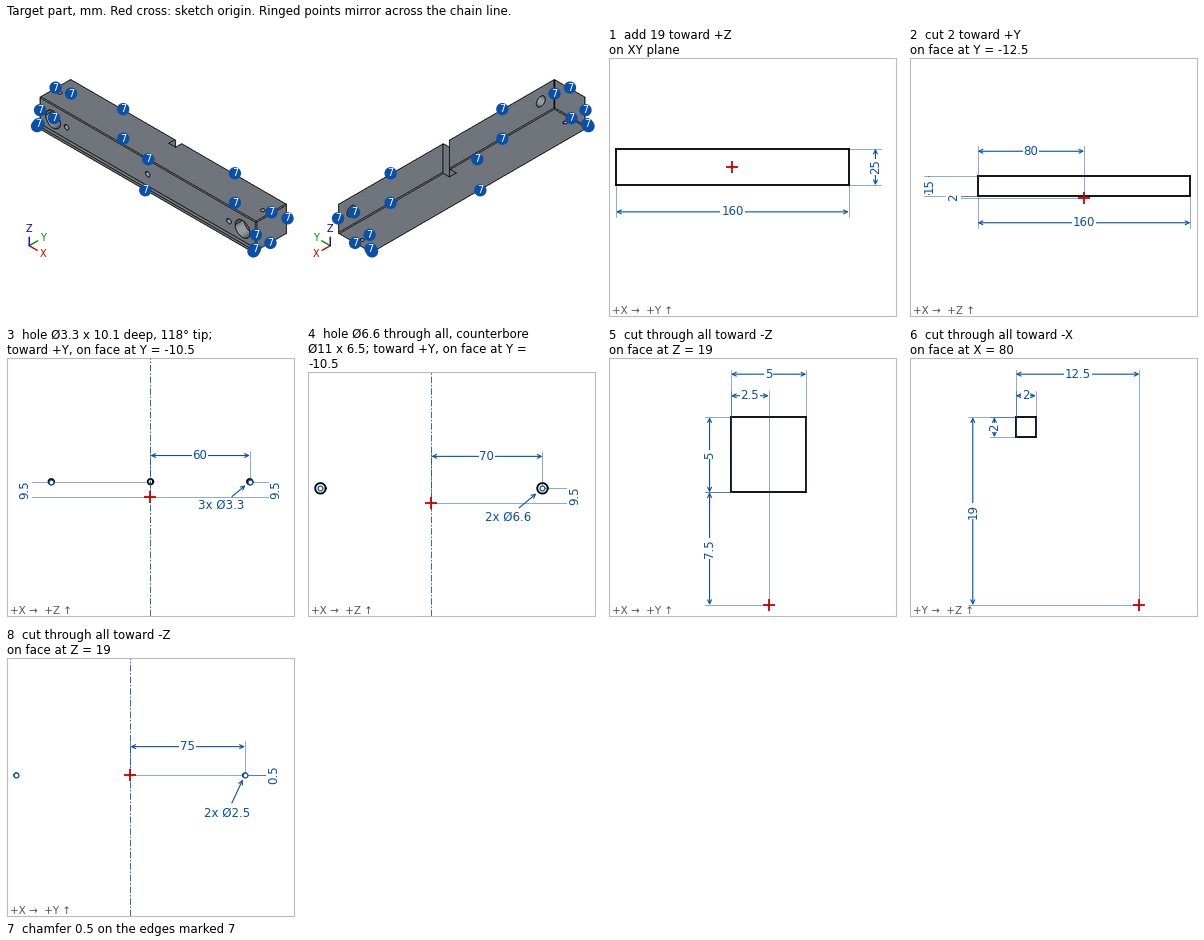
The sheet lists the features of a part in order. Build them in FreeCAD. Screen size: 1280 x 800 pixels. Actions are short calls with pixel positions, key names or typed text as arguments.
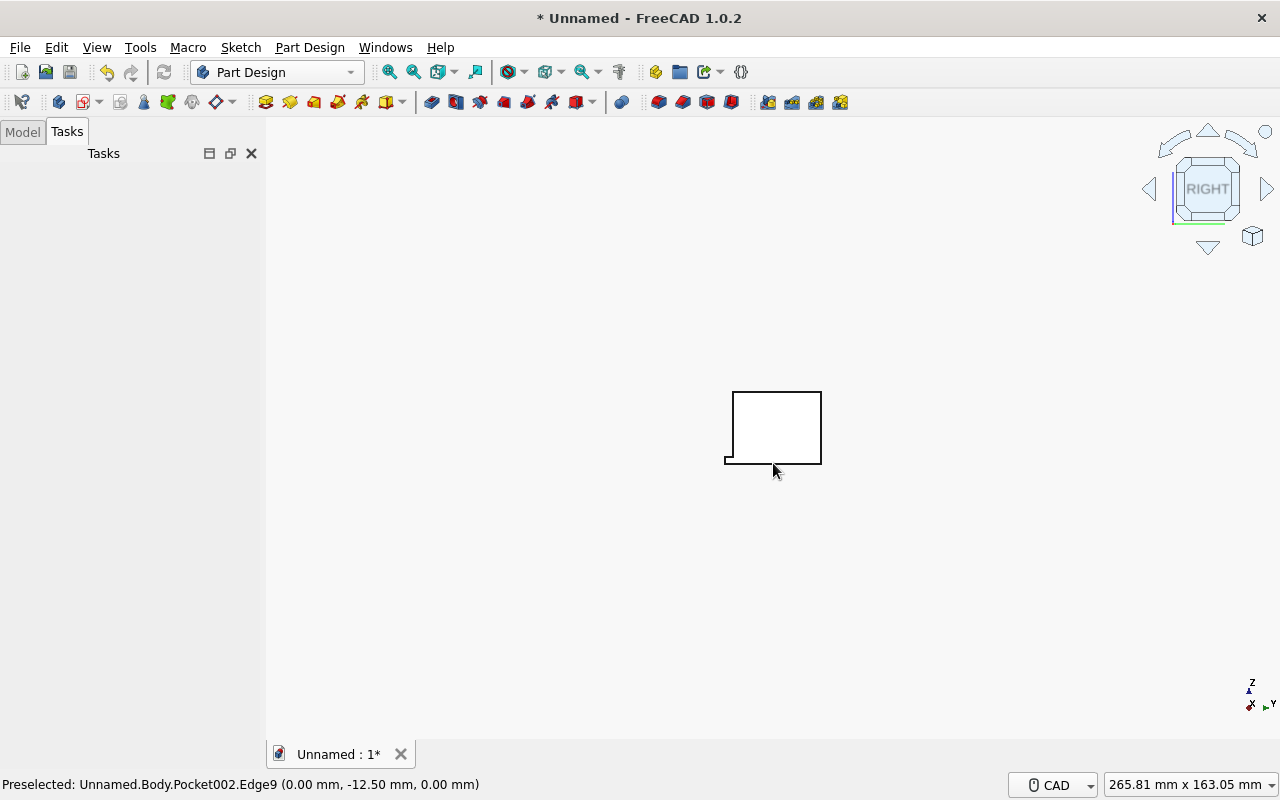
click(390, 72)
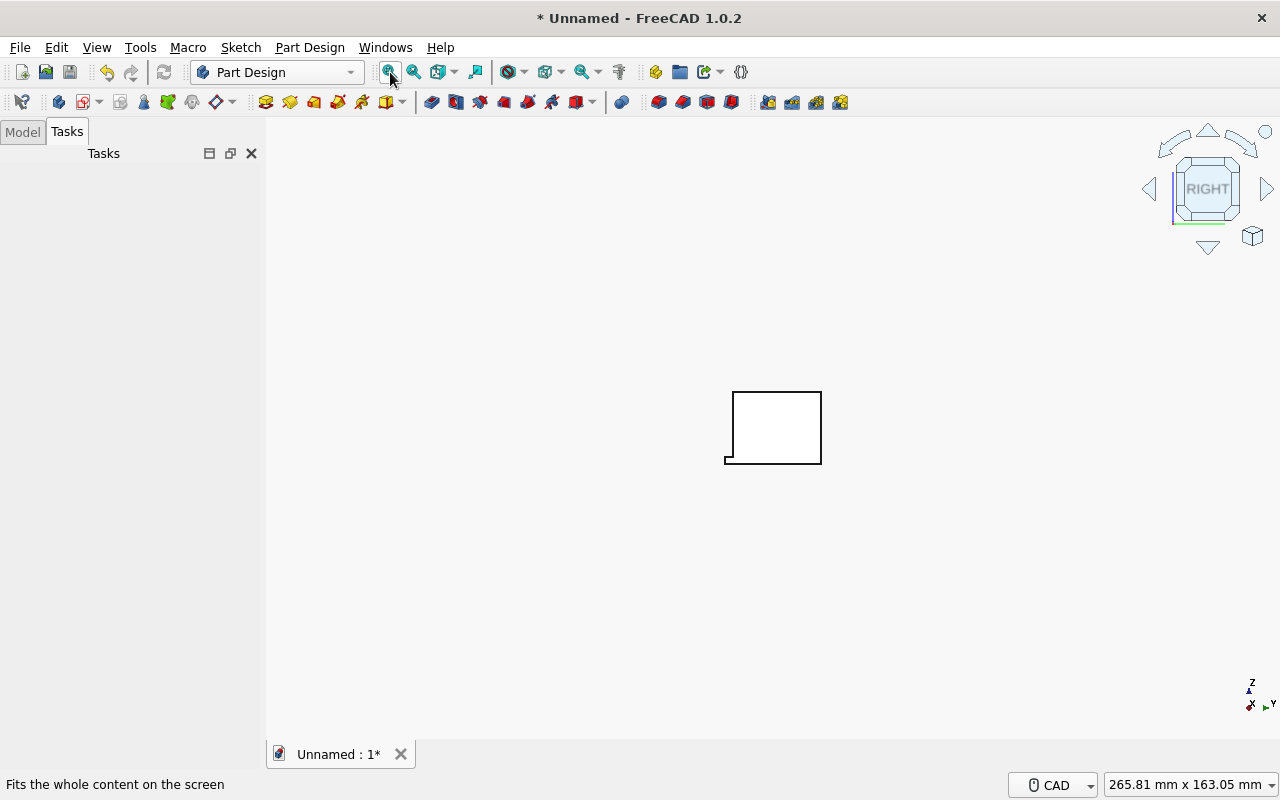
key(5)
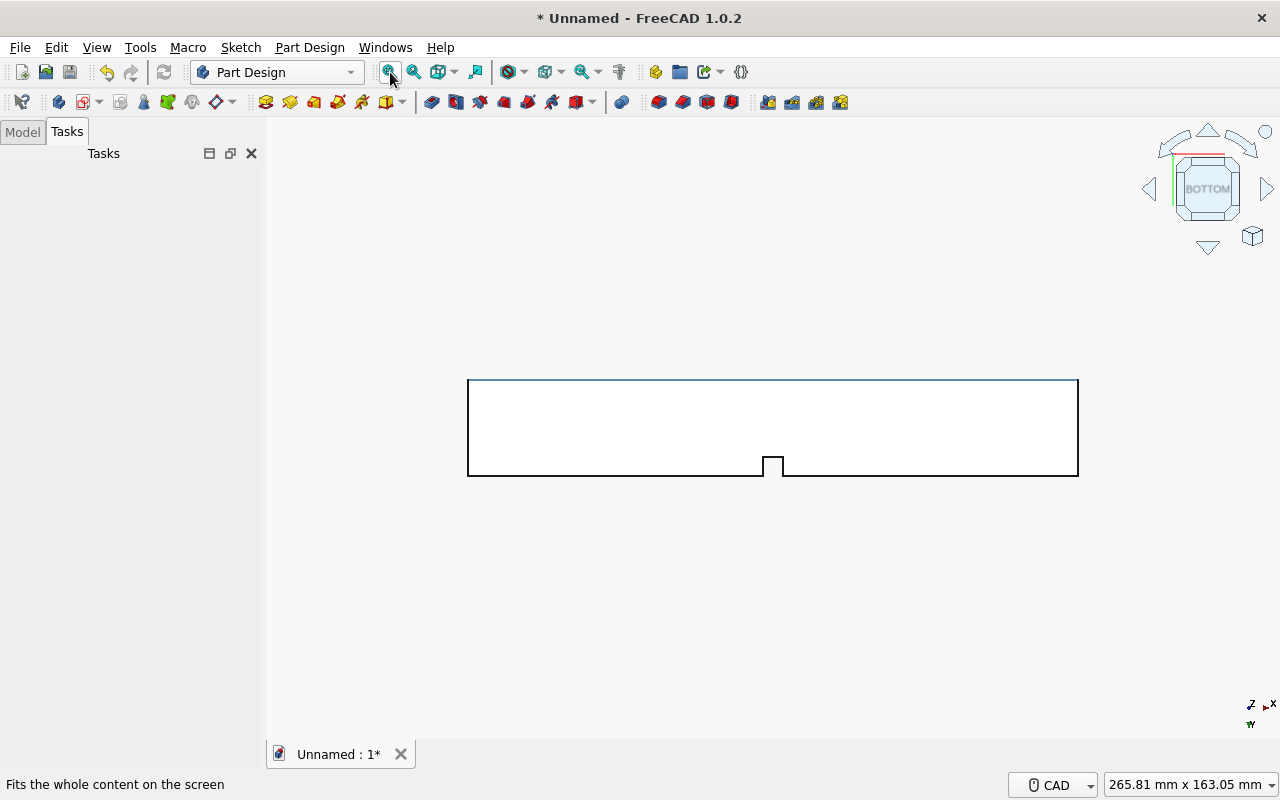
click(930, 475, ctrl)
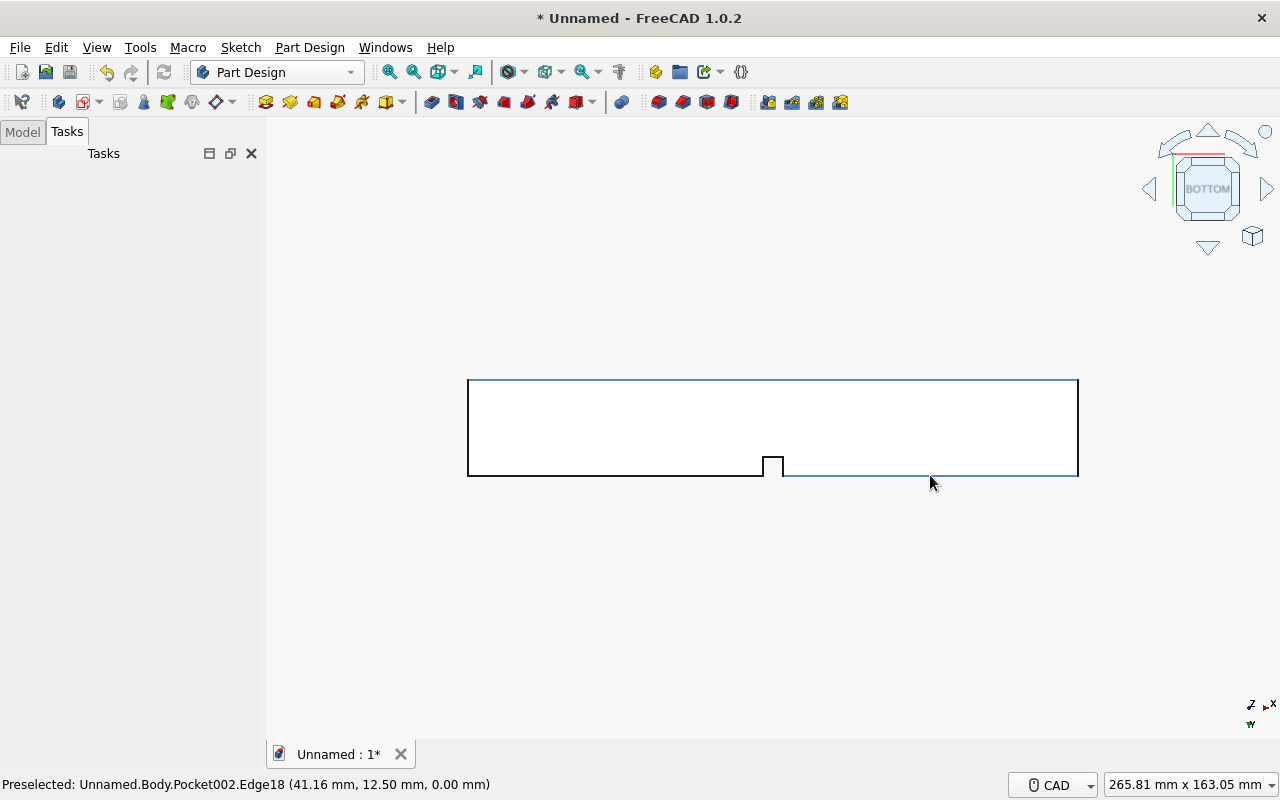
click(616, 475, ctrl)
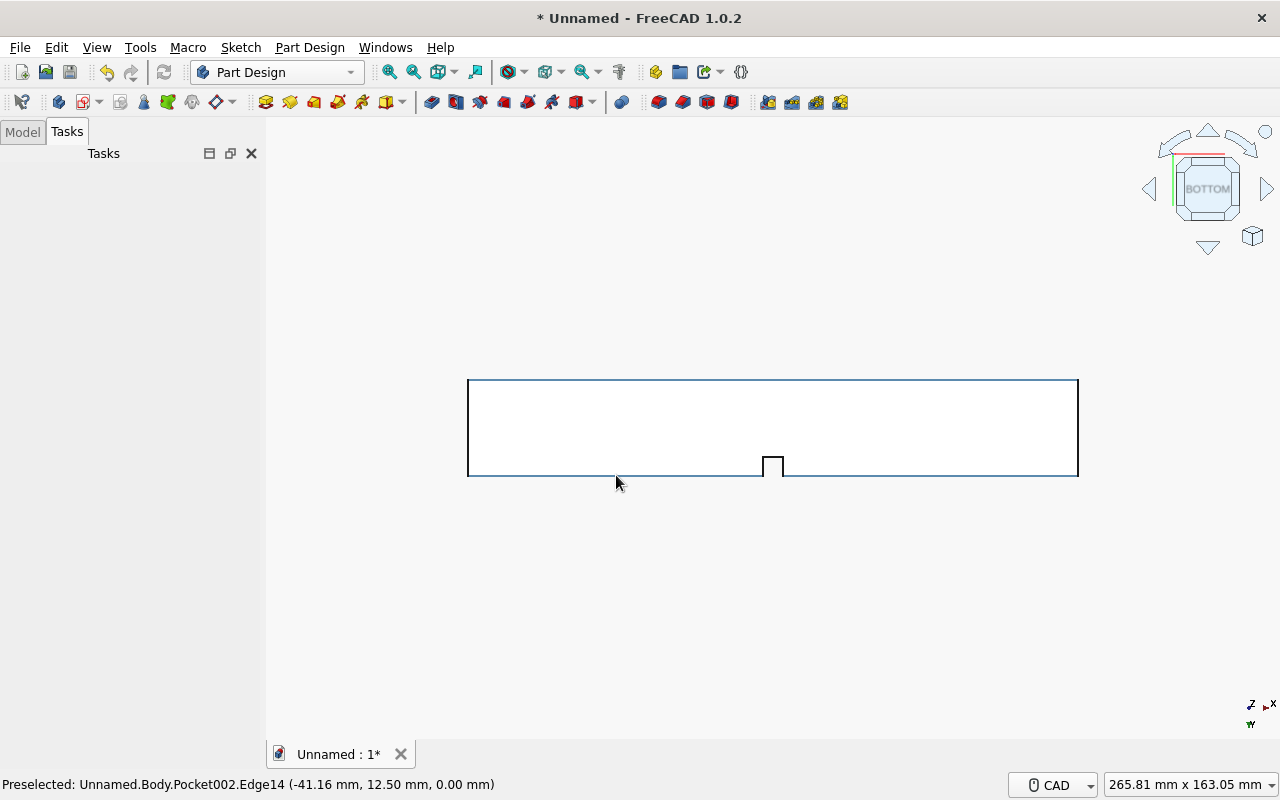
key(4)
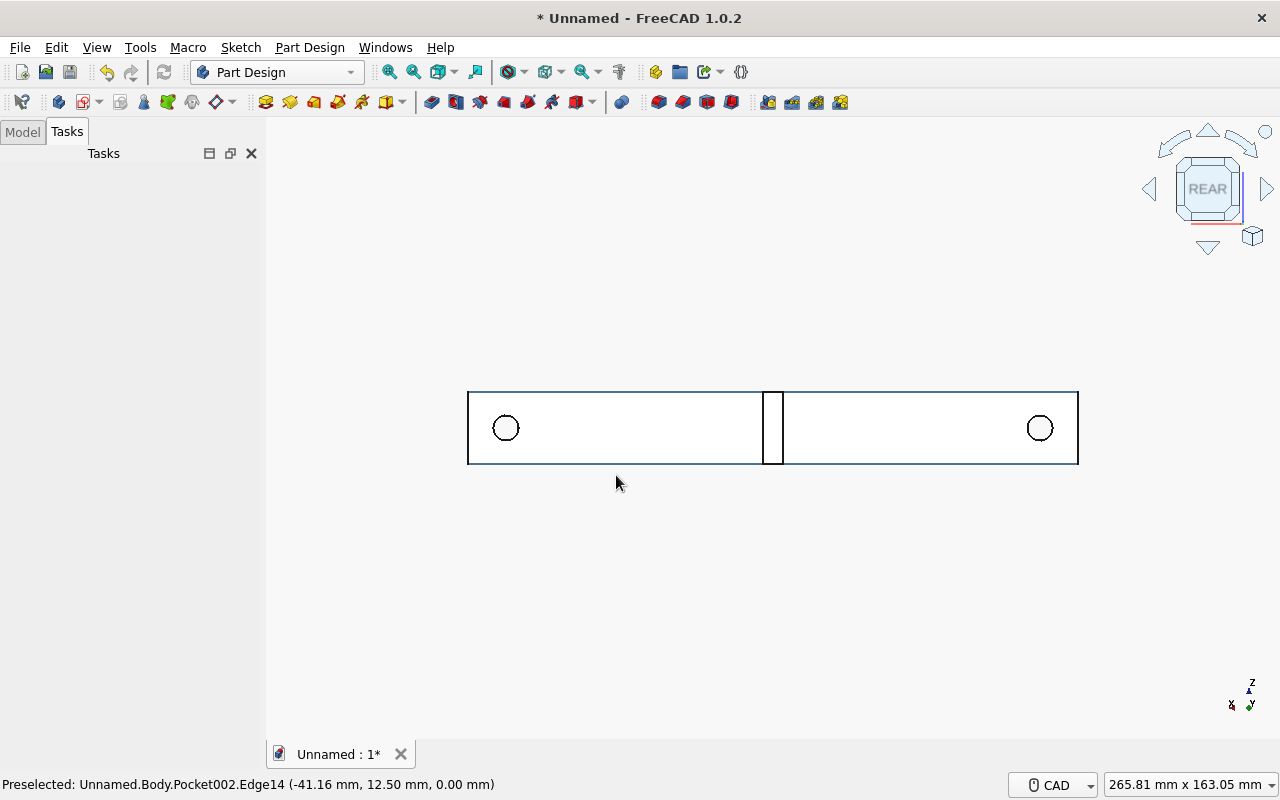
key(6)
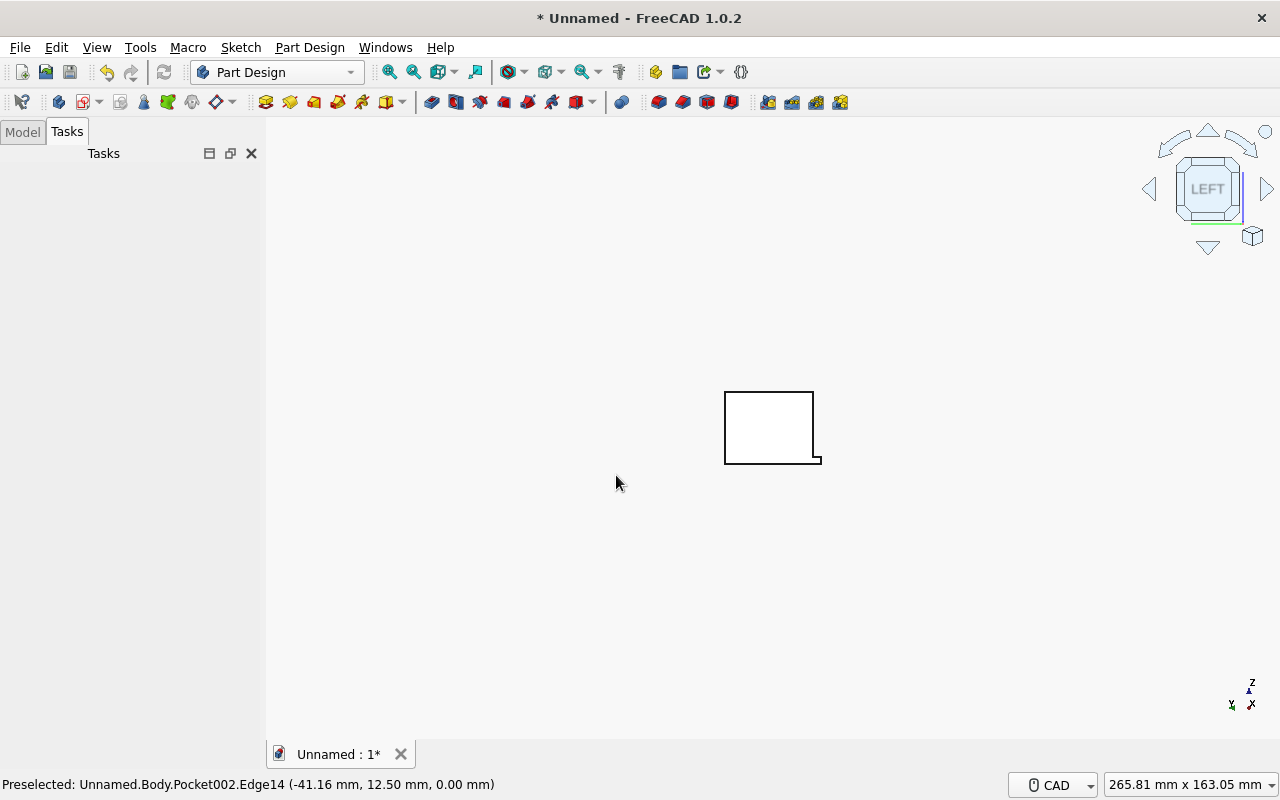
click(390, 72)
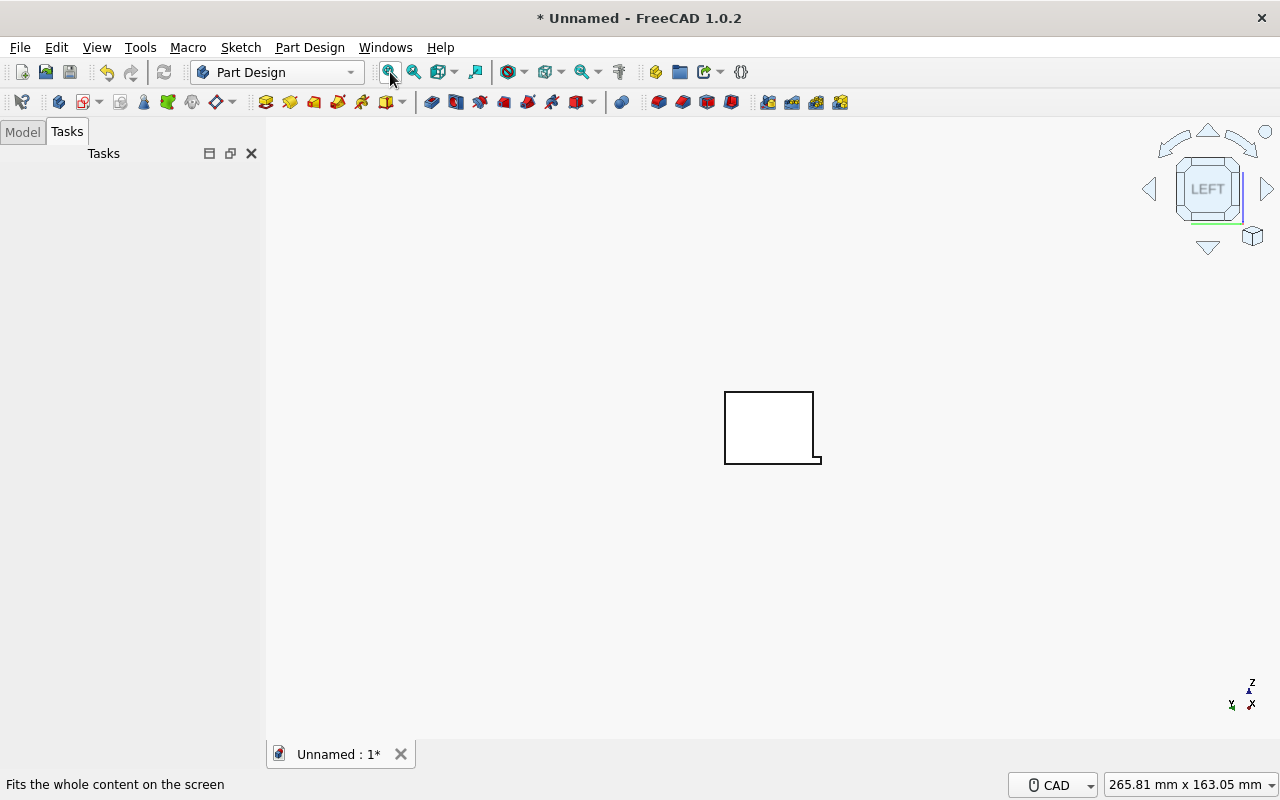
click(773, 427, ctrl)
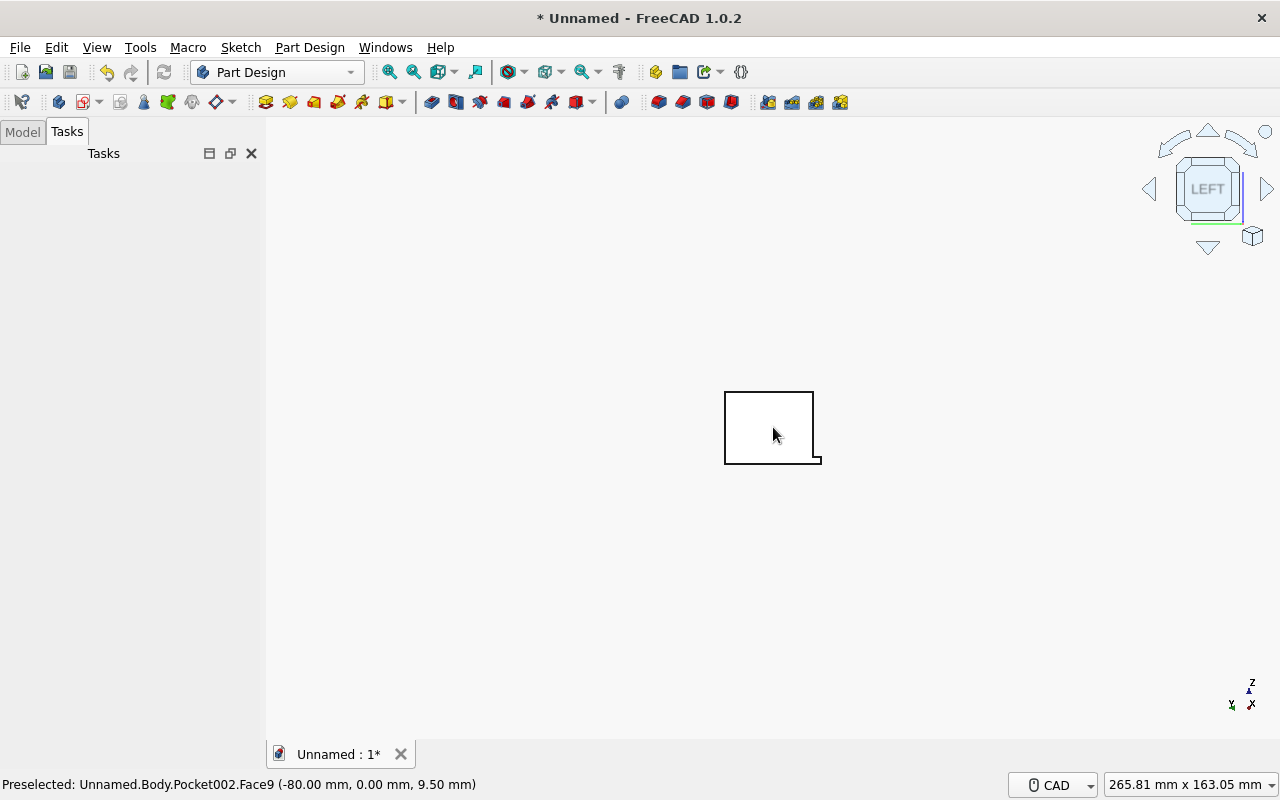
click(684, 102)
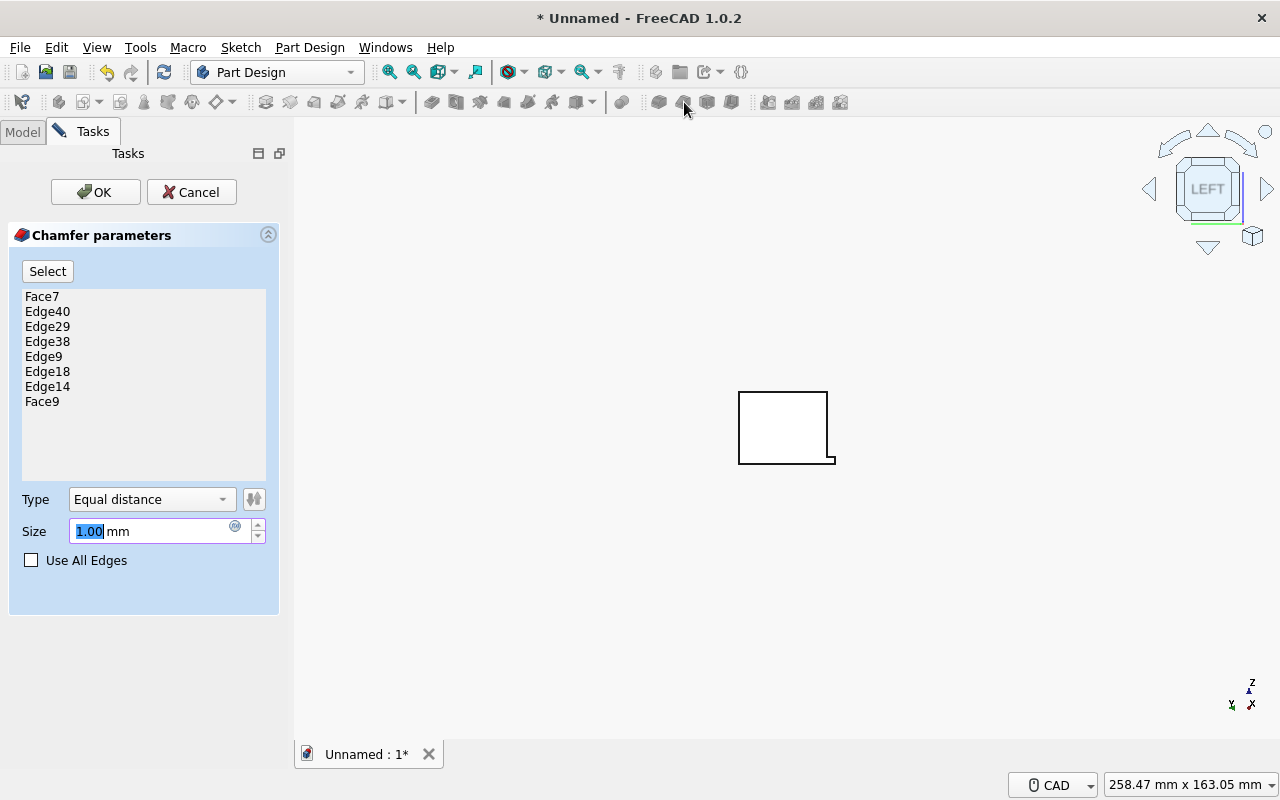
text(0.5)
key(Tab)